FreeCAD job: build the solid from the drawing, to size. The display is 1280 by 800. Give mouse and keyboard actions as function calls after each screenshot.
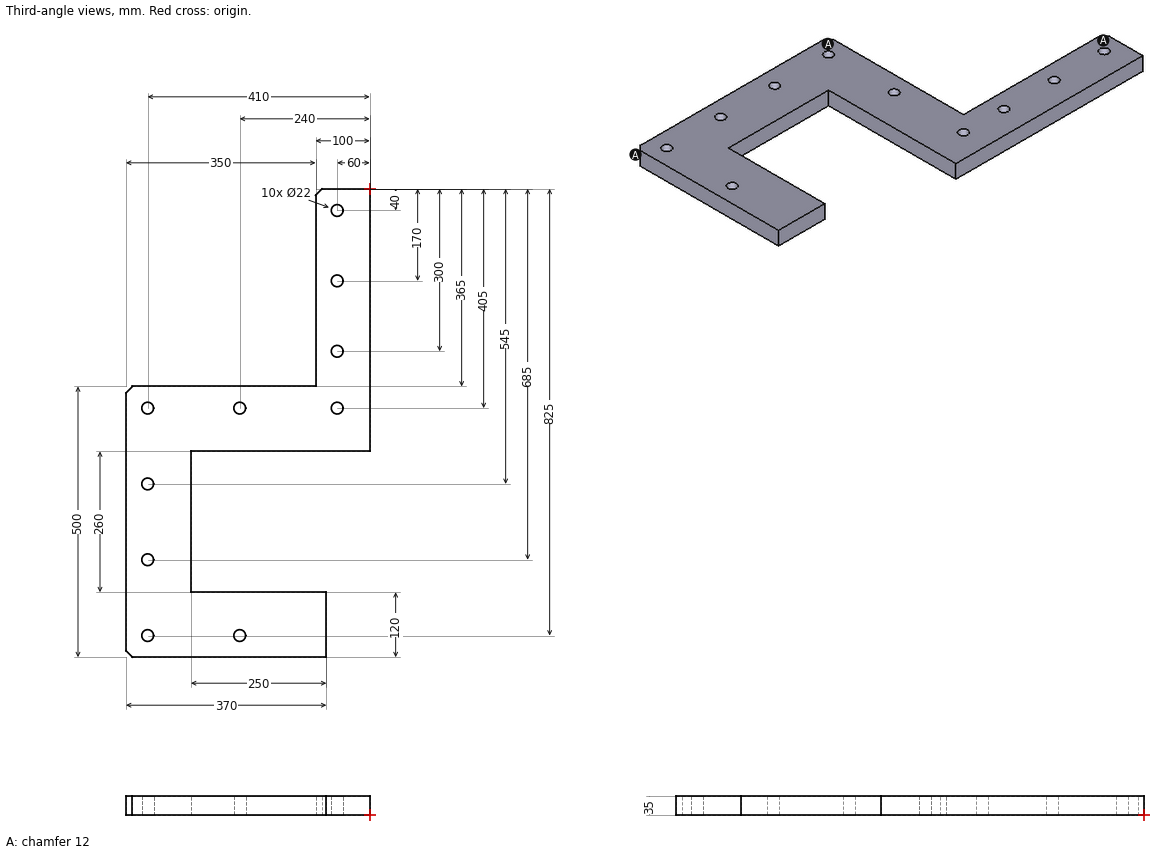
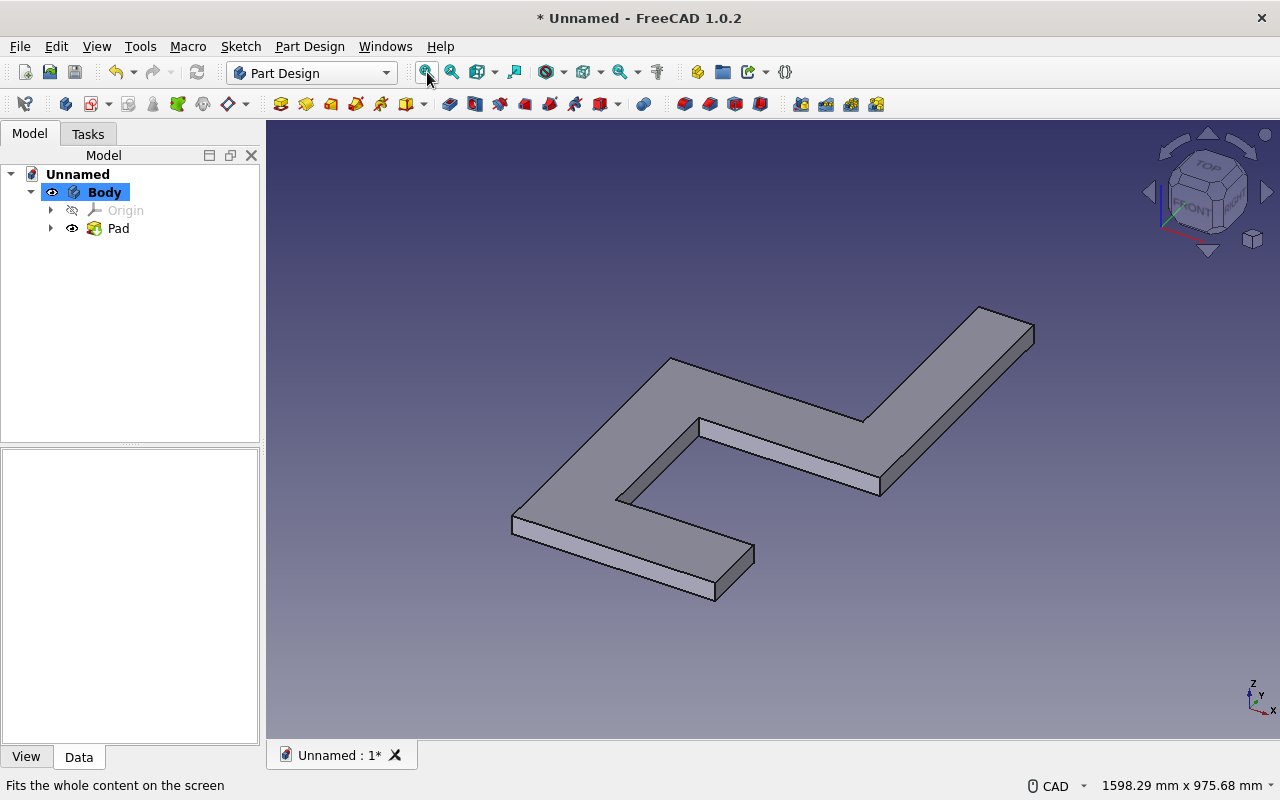
key(0)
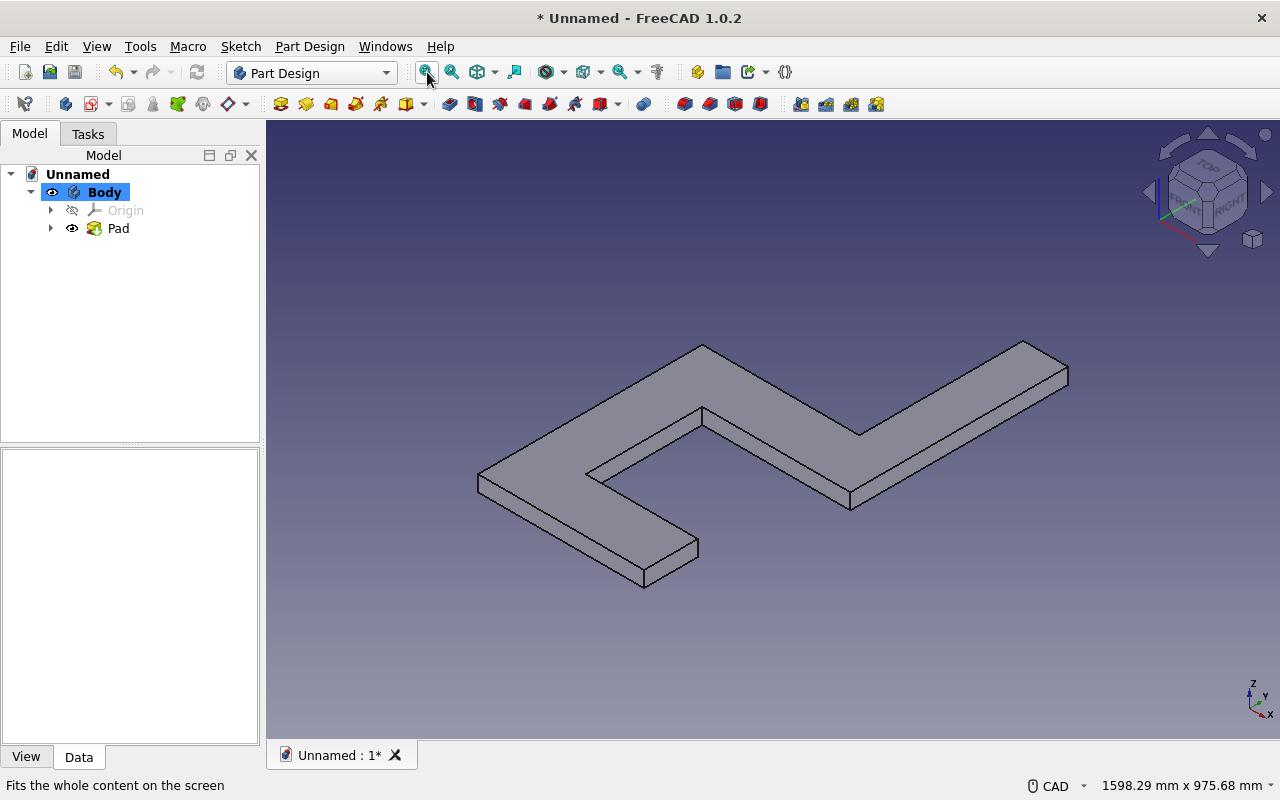
key(2)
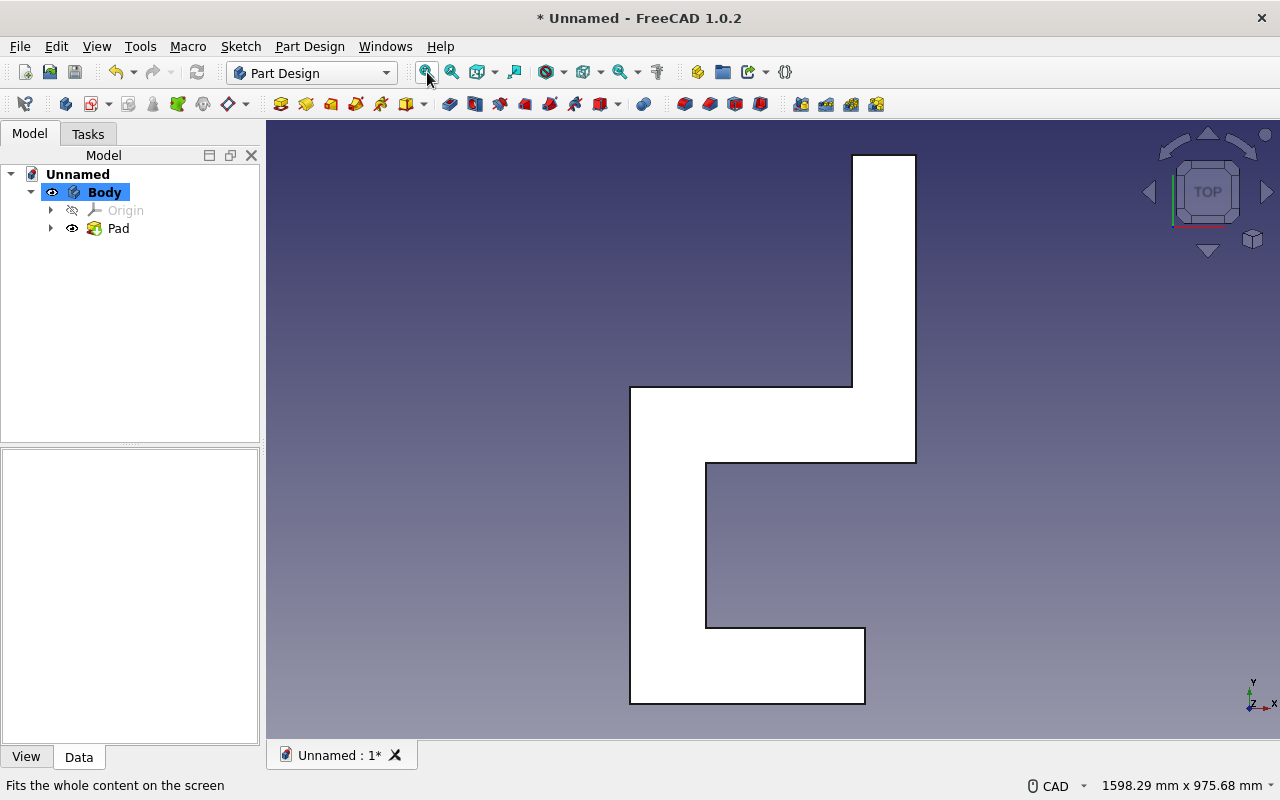
key(1)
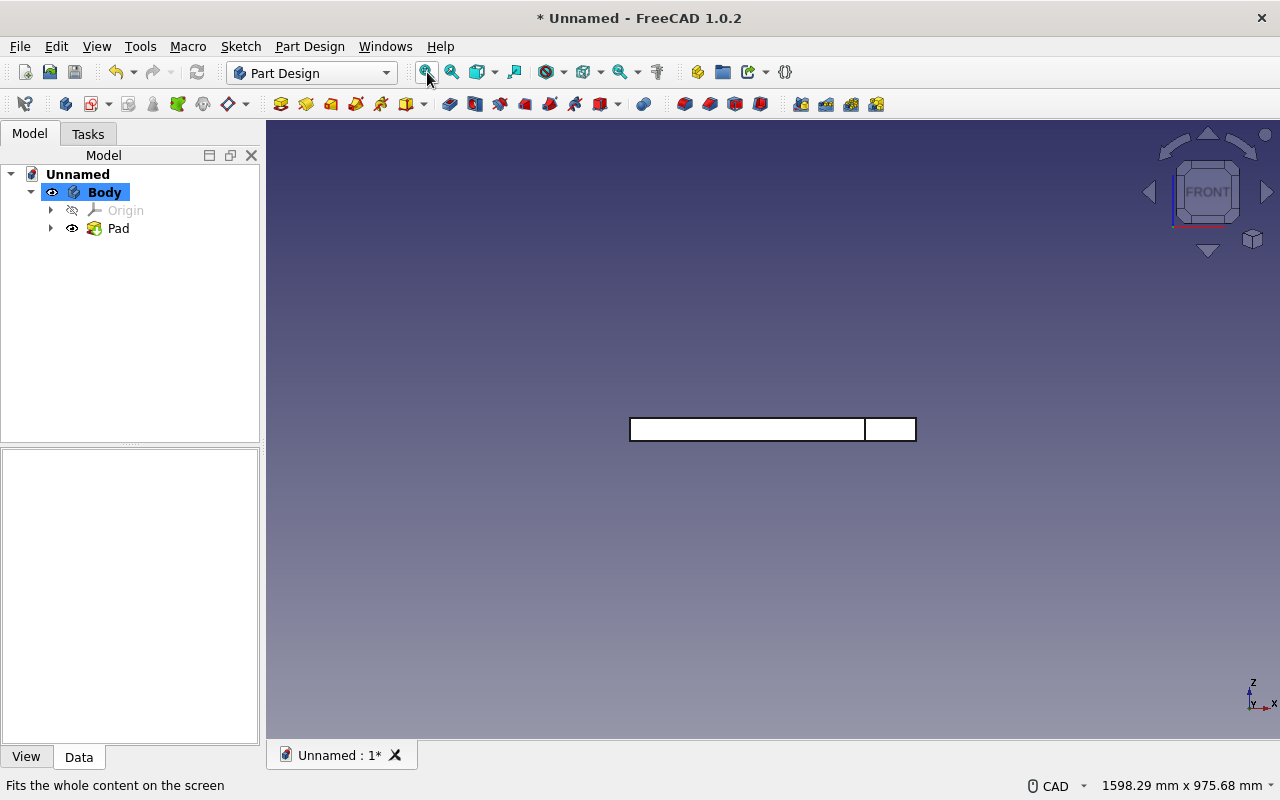
click(427, 72)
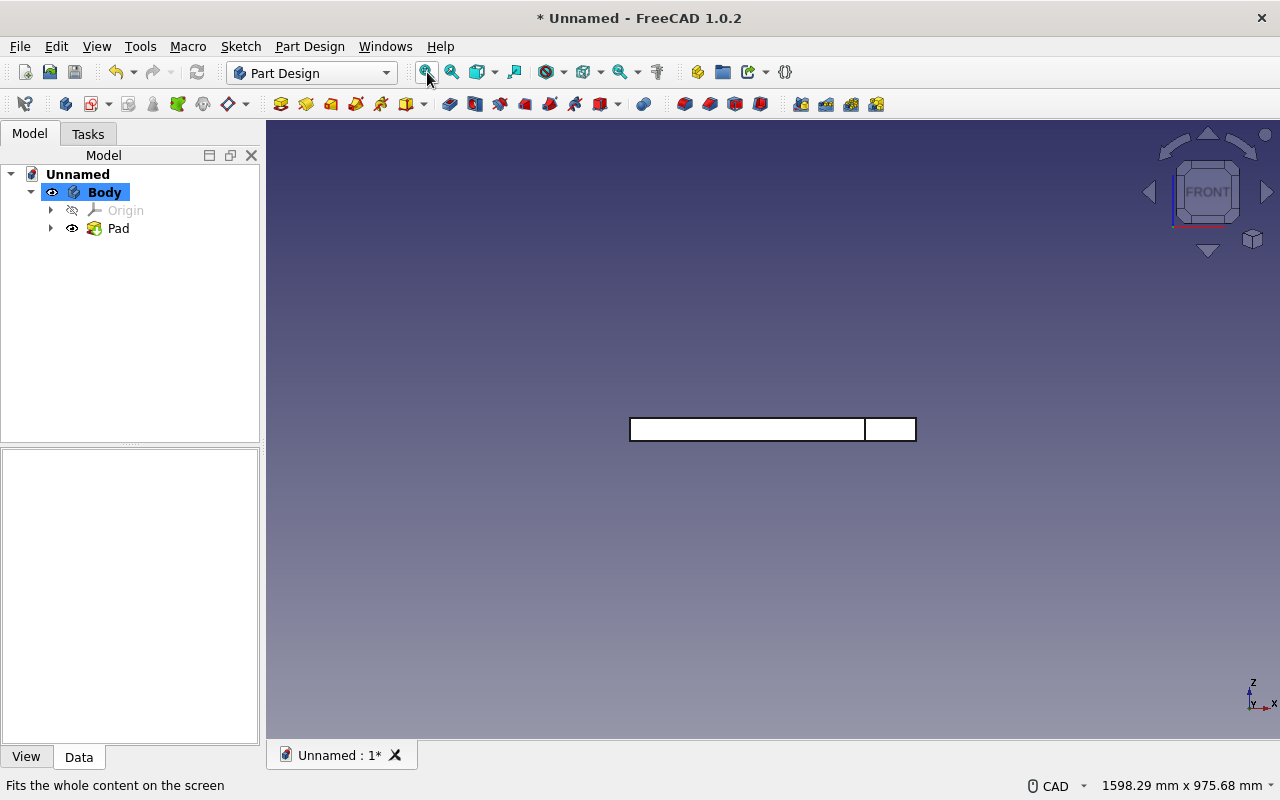
click(630, 429)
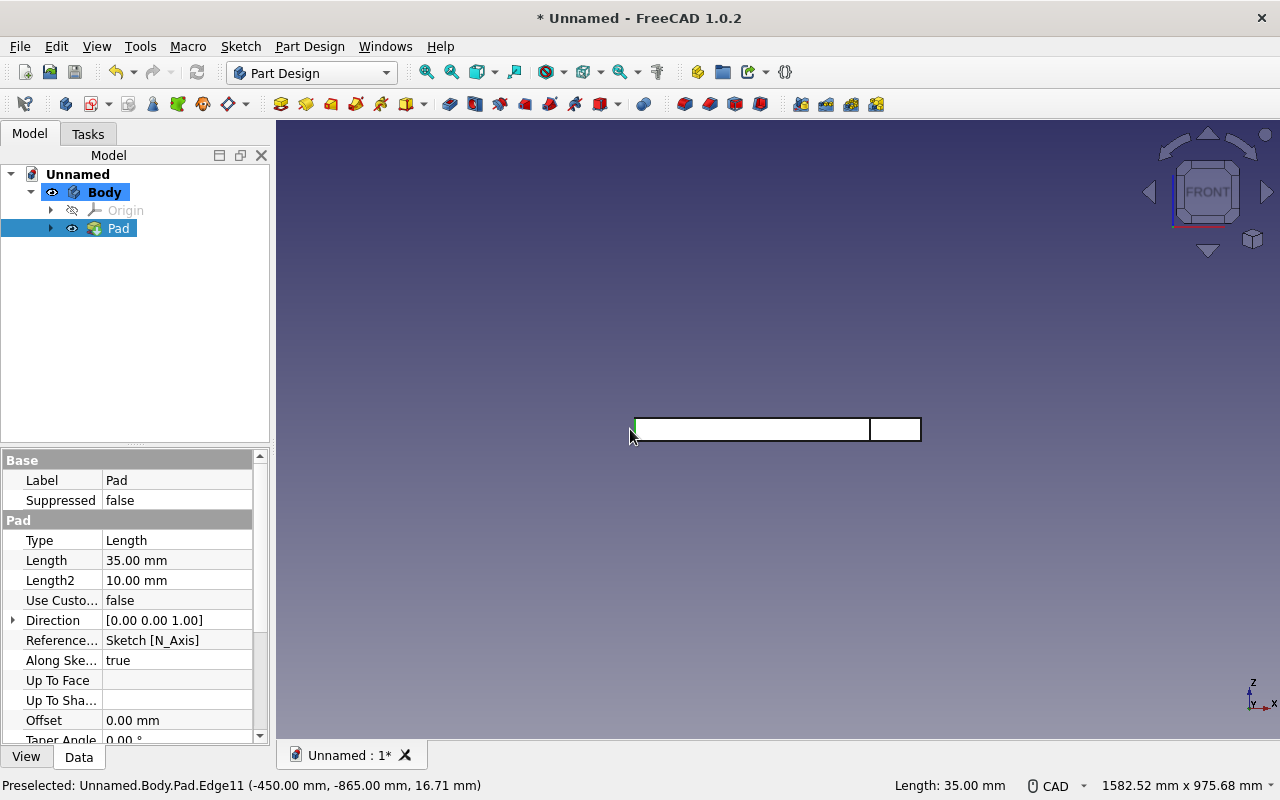
key(3)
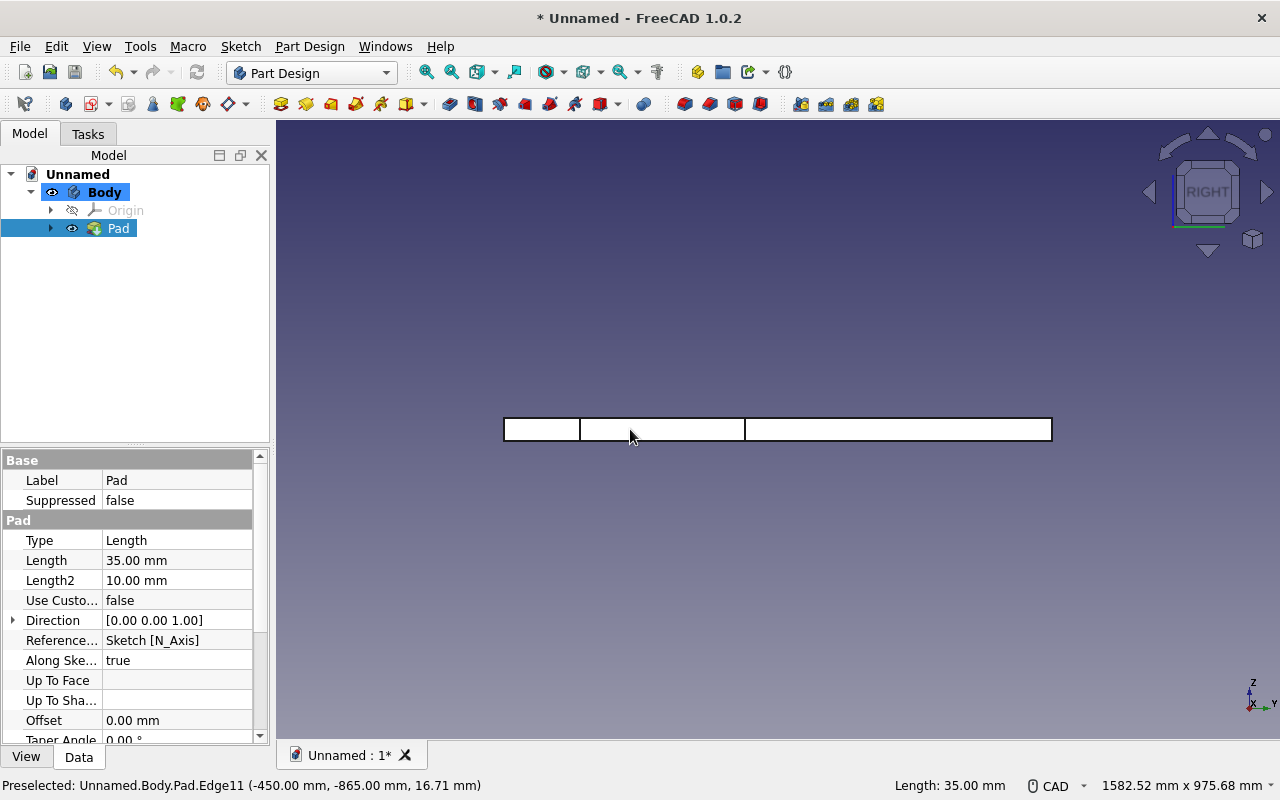
key(5)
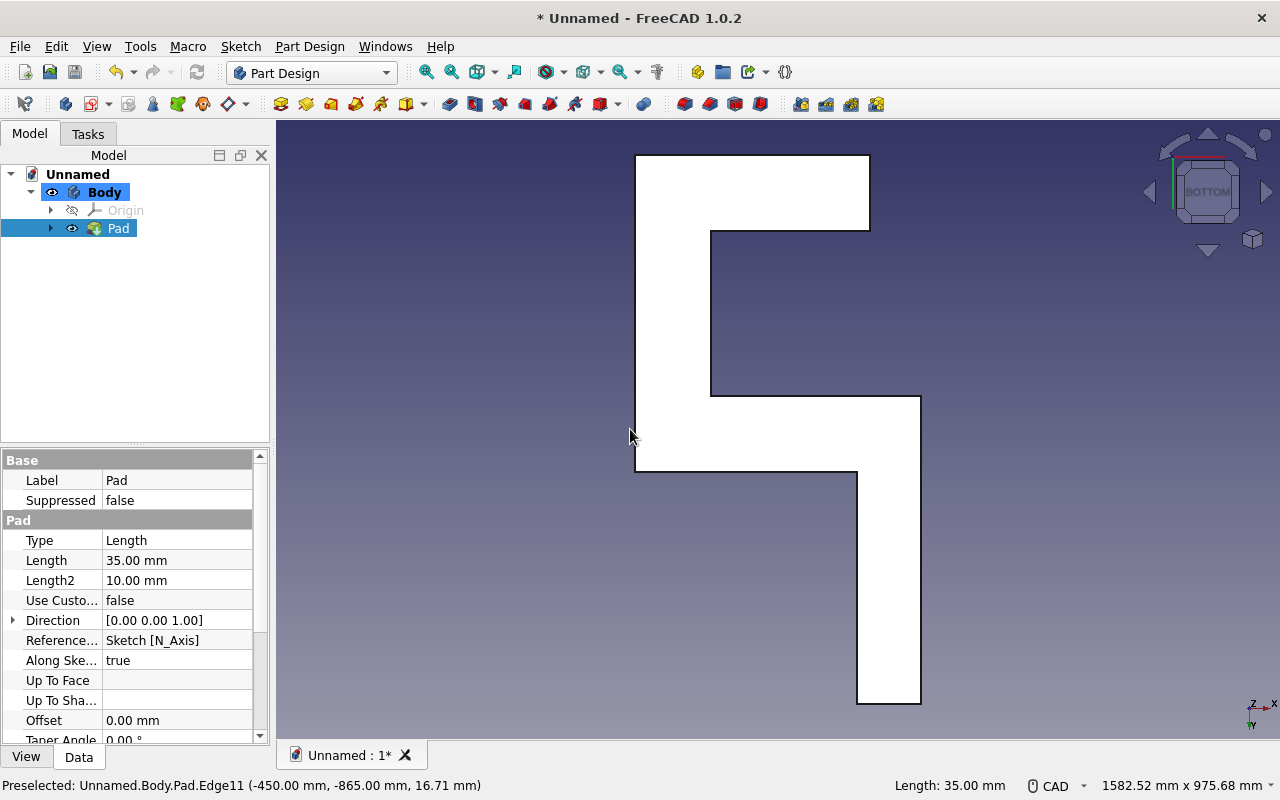
key(4)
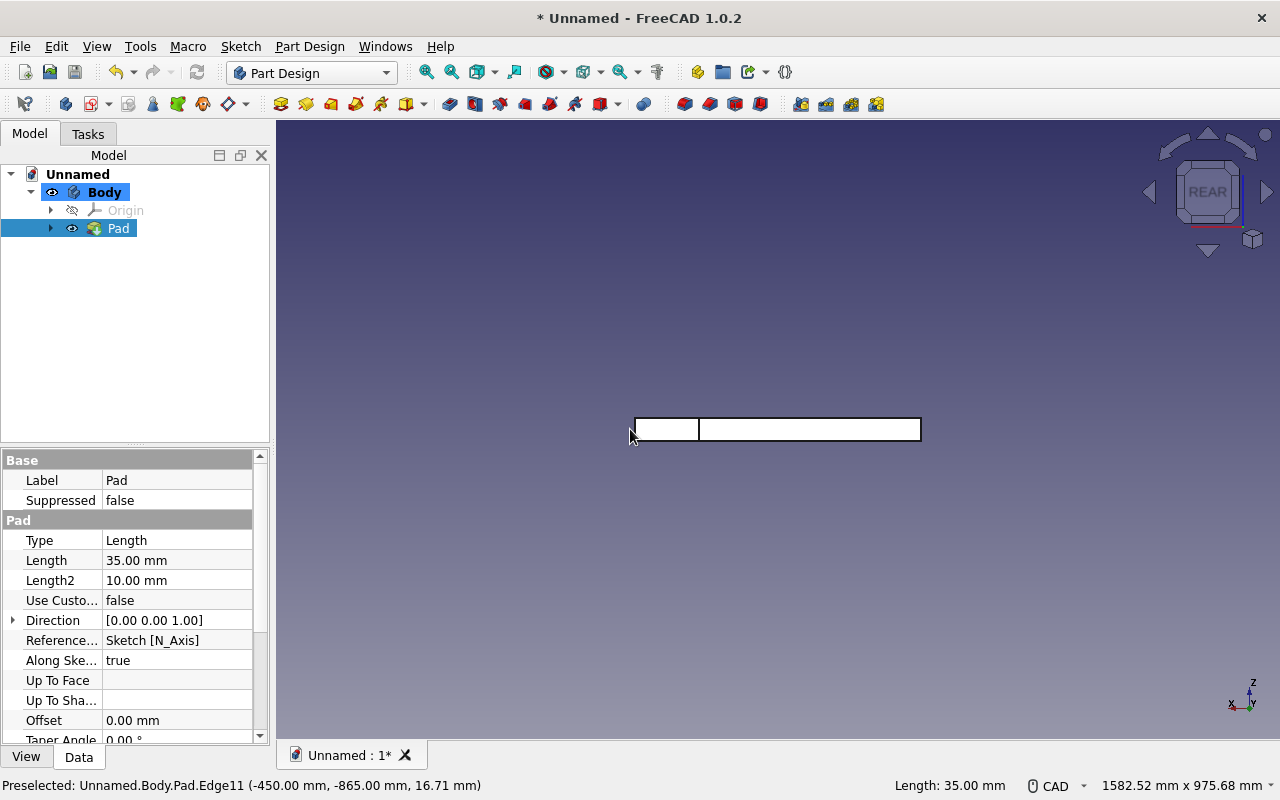
click(427, 72)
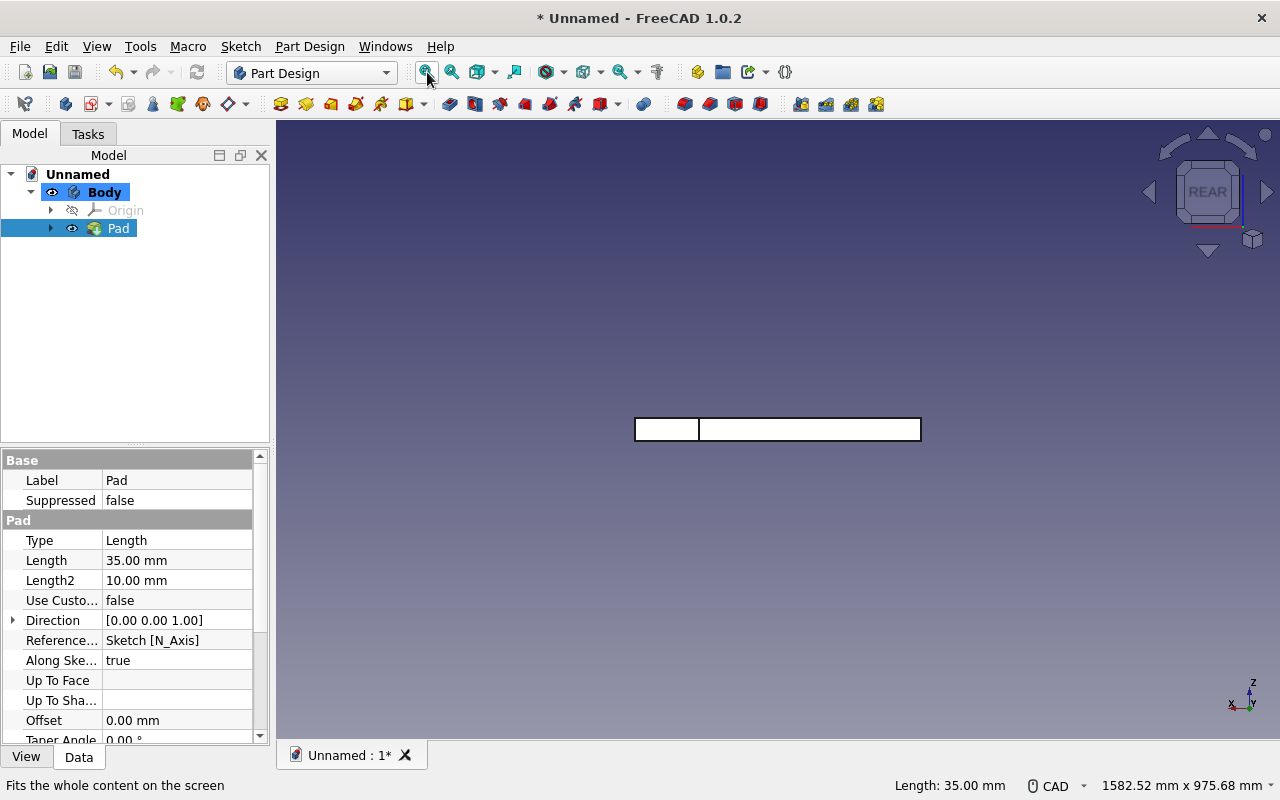
click(699, 429, ctrl)